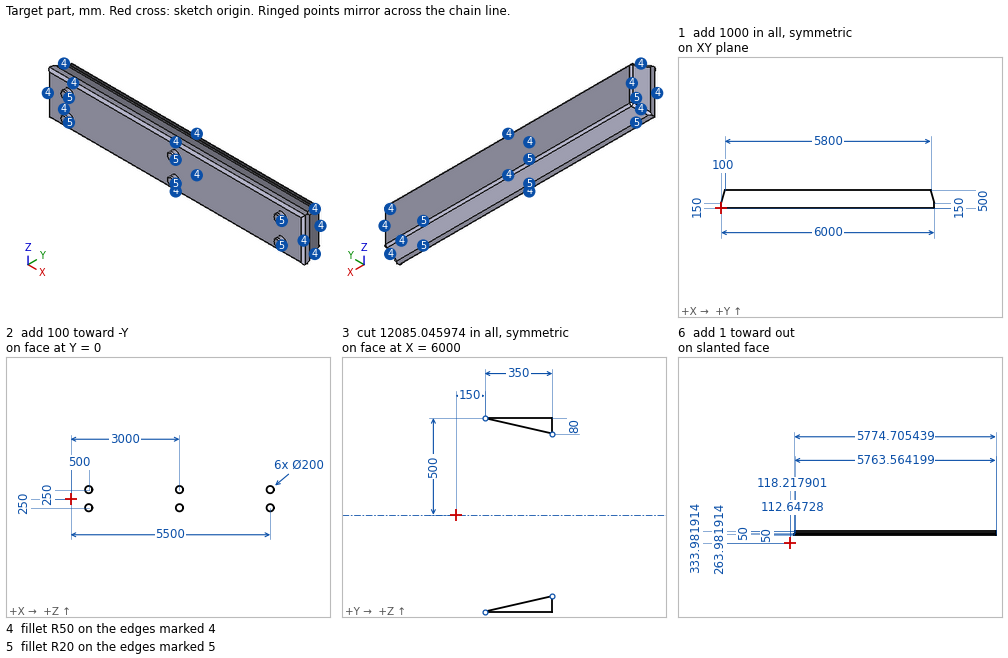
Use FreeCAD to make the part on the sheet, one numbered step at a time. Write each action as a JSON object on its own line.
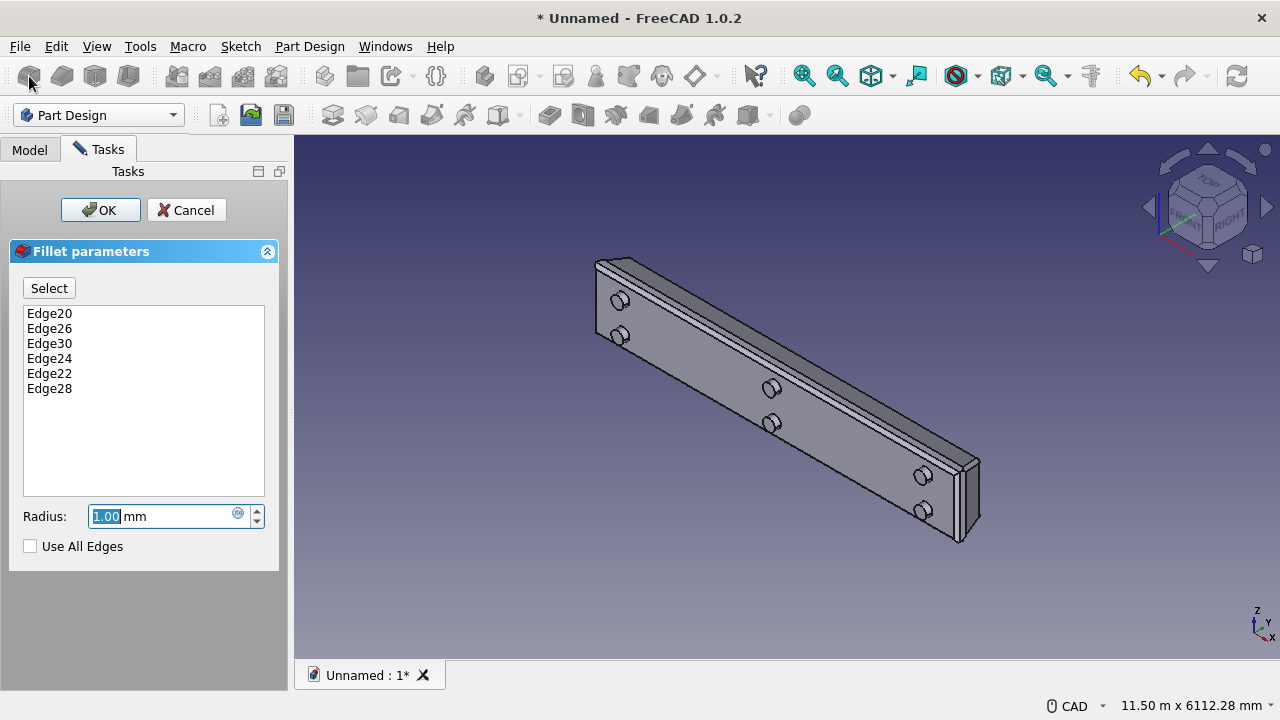
{"action": "type", "text": "20"}
{"action": "key", "text": "Tab"}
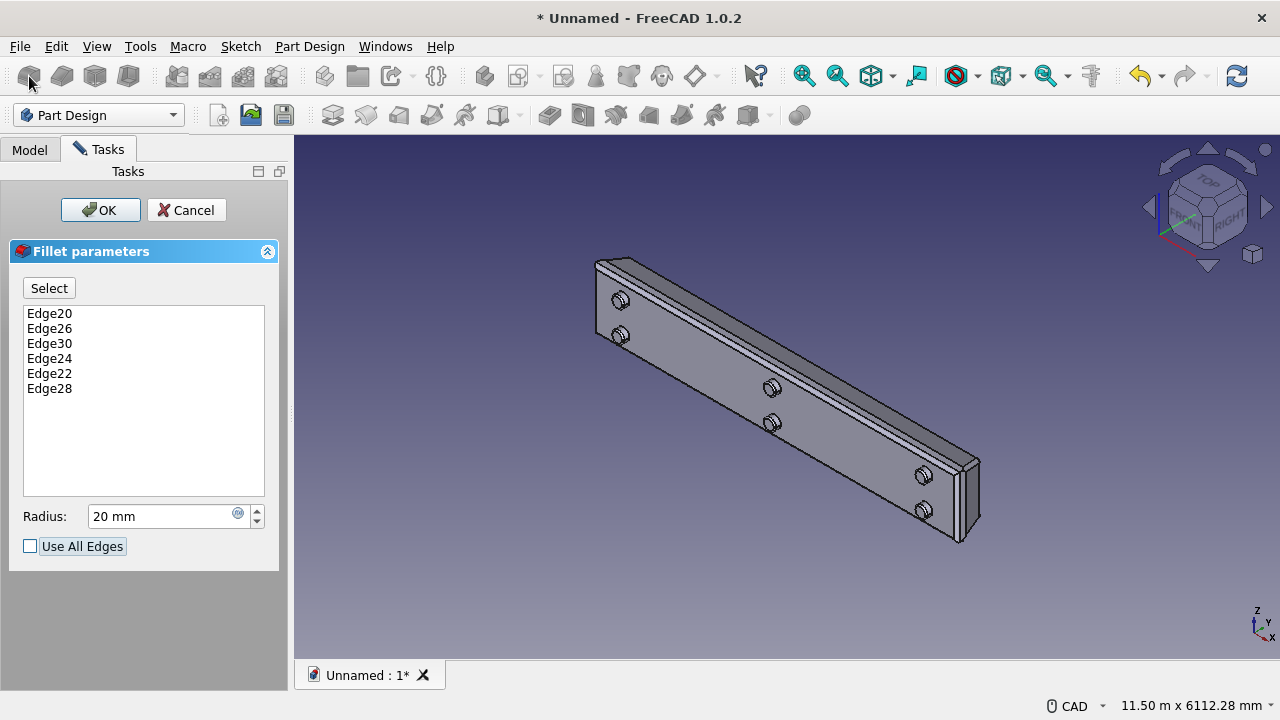
{"action": "left_click", "coordinate": [101, 210]}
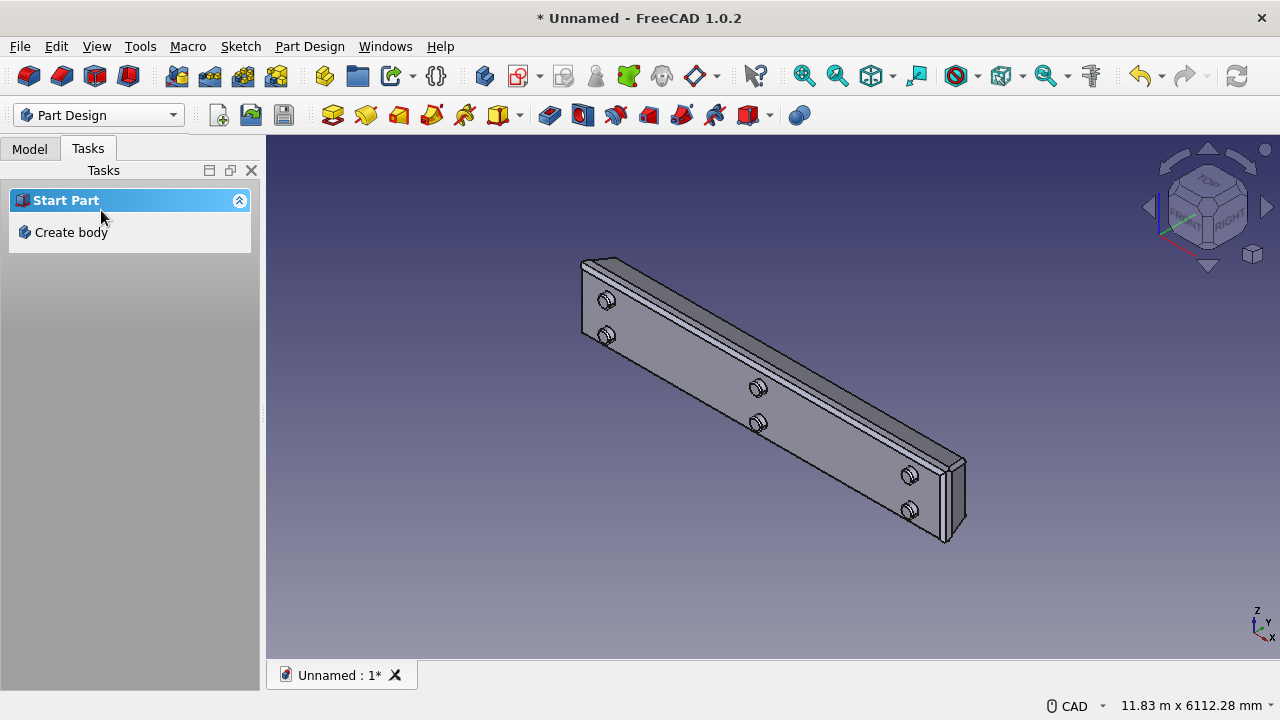
{"action": "key", "text": "2"}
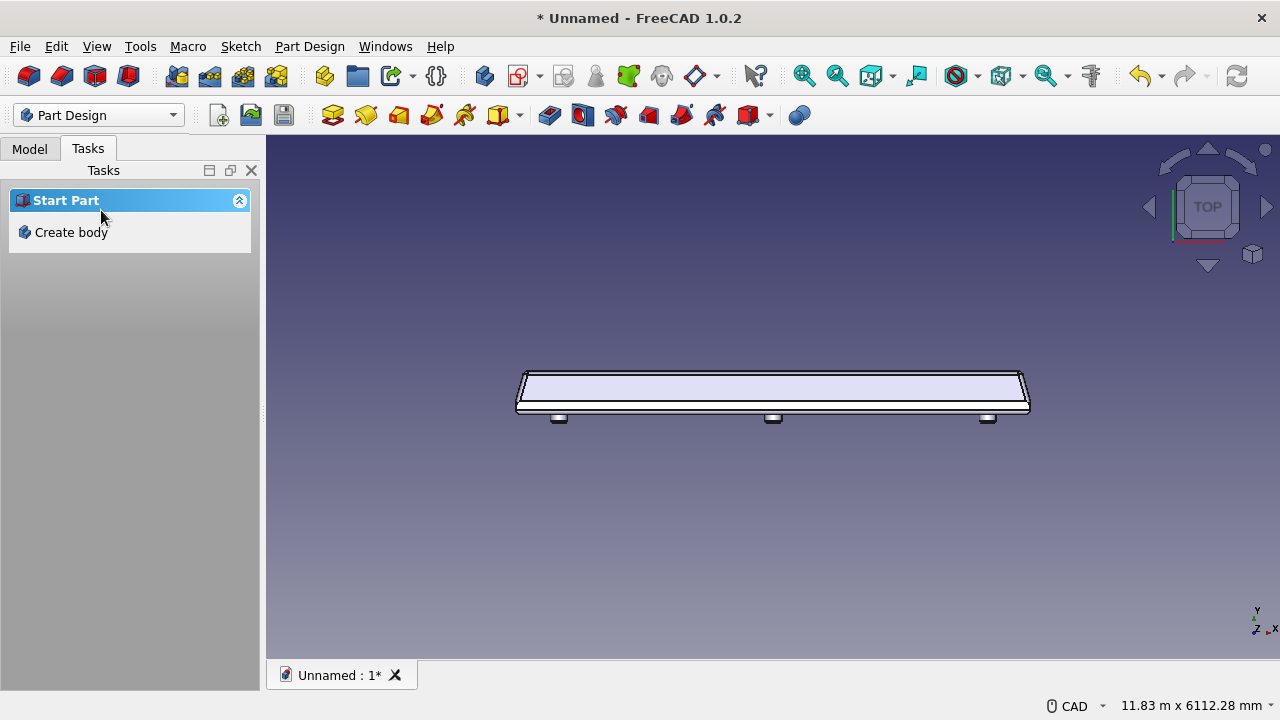
{"action": "left_click", "coordinate": [990, 387]}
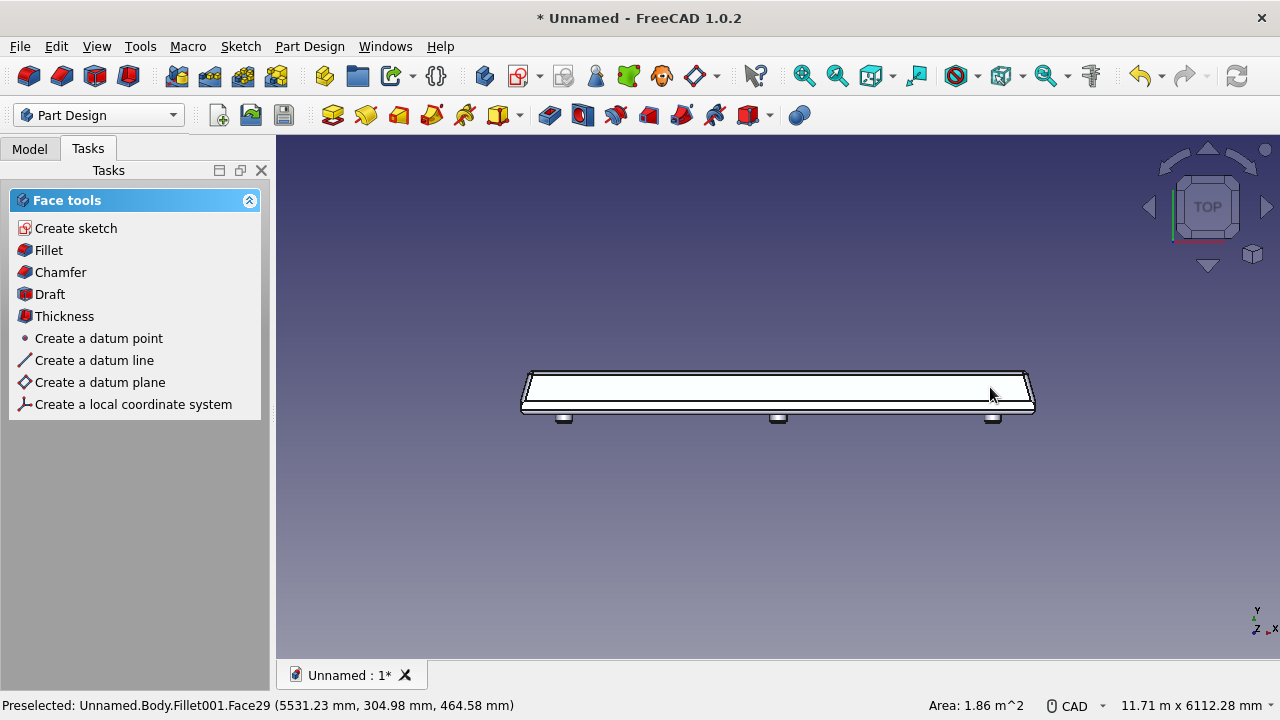
{"action": "left_click", "coordinate": [518, 76]}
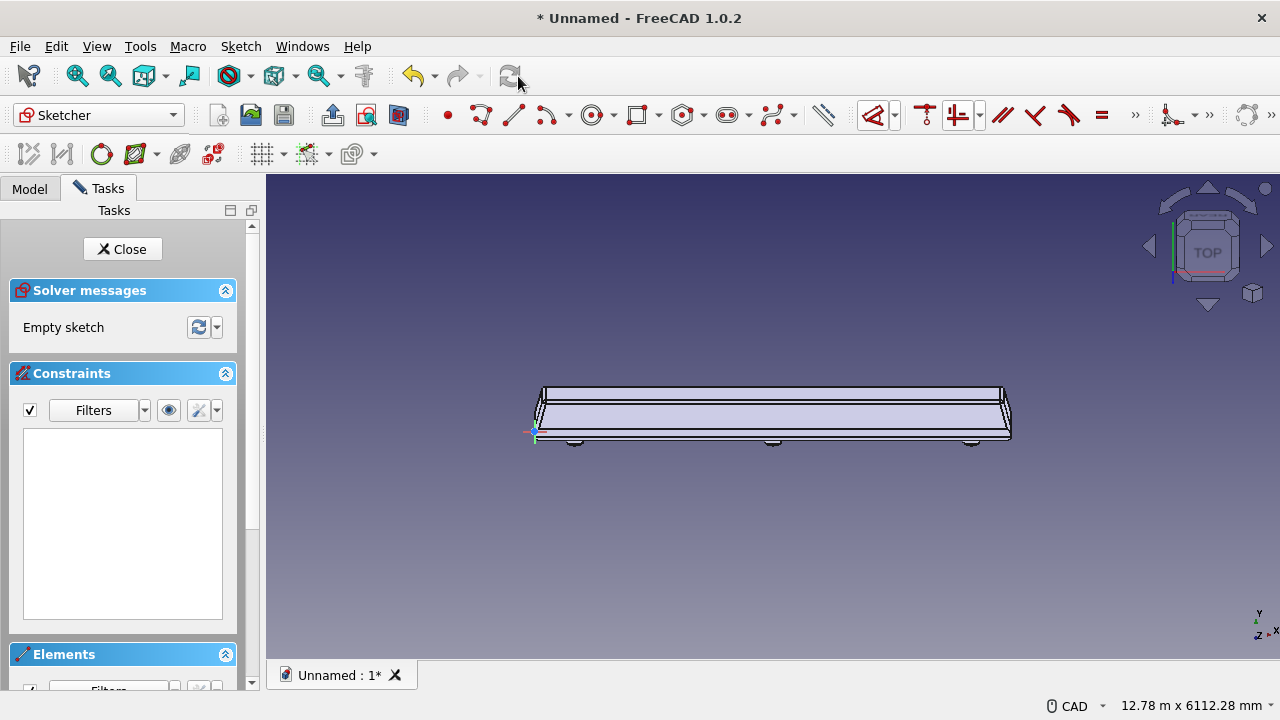
{"action": "left_click", "coordinate": [636, 116]}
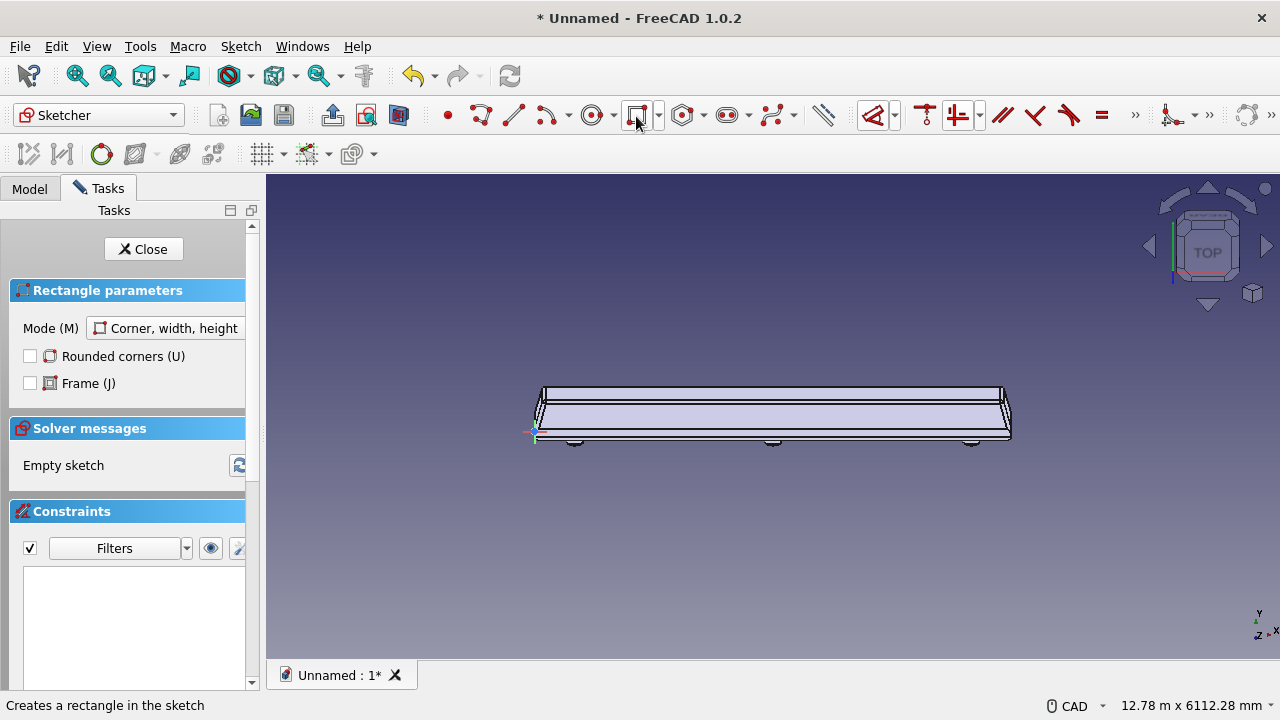
{"action": "scroll", "coordinate": [544, 405], "scroll_direction": "up", "scroll_amount": 7}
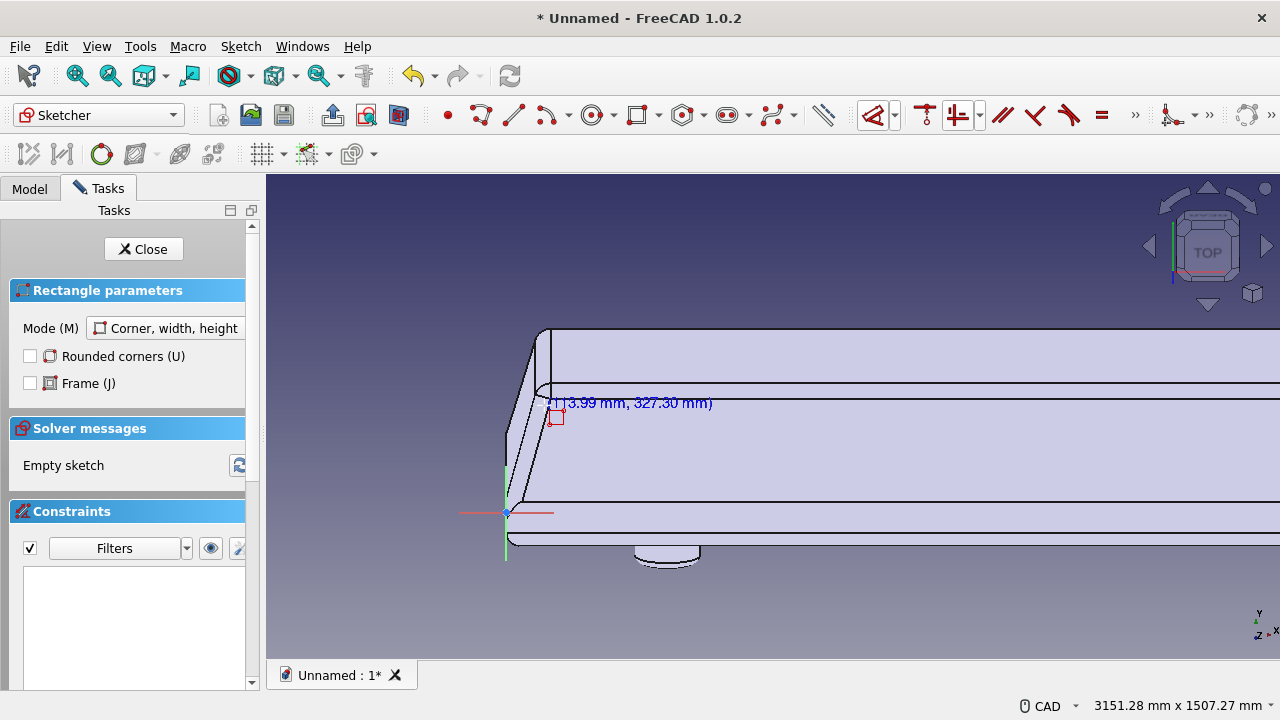
{"action": "left_click", "coordinate": [545, 405]}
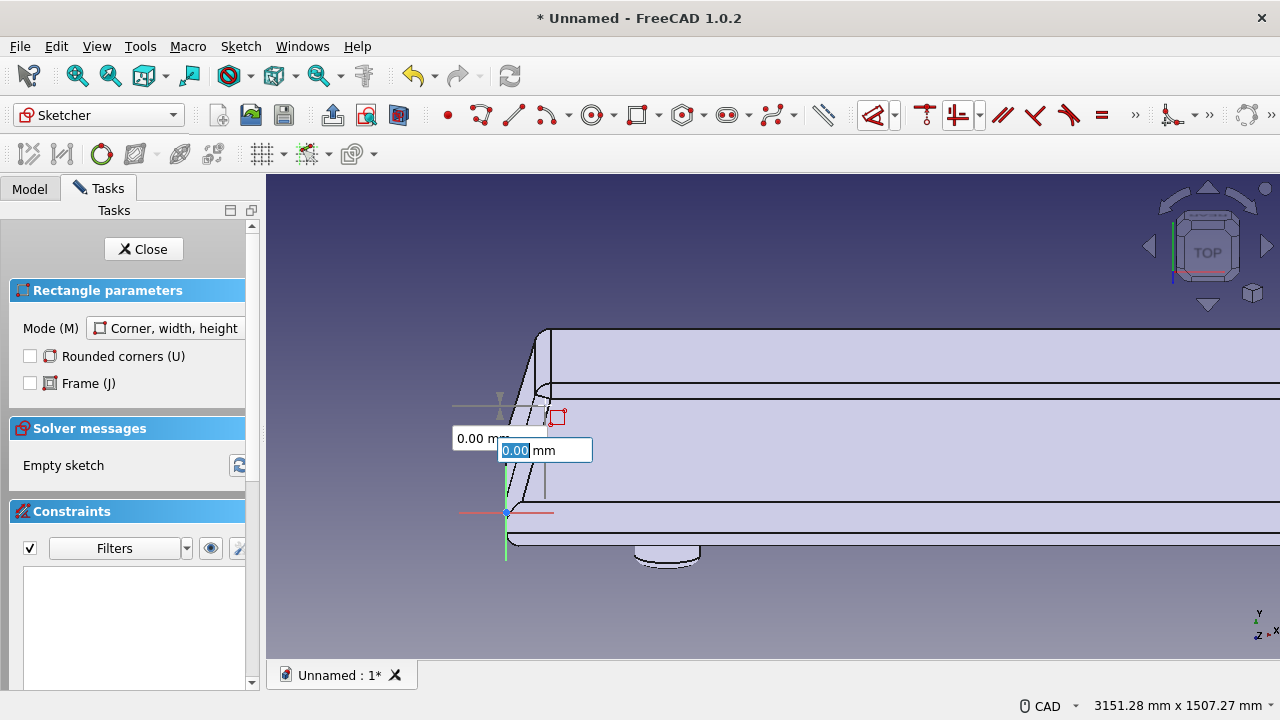
{"action": "scroll", "coordinate": [382, 398], "scroll_direction": "down", "scroll_amount": 6}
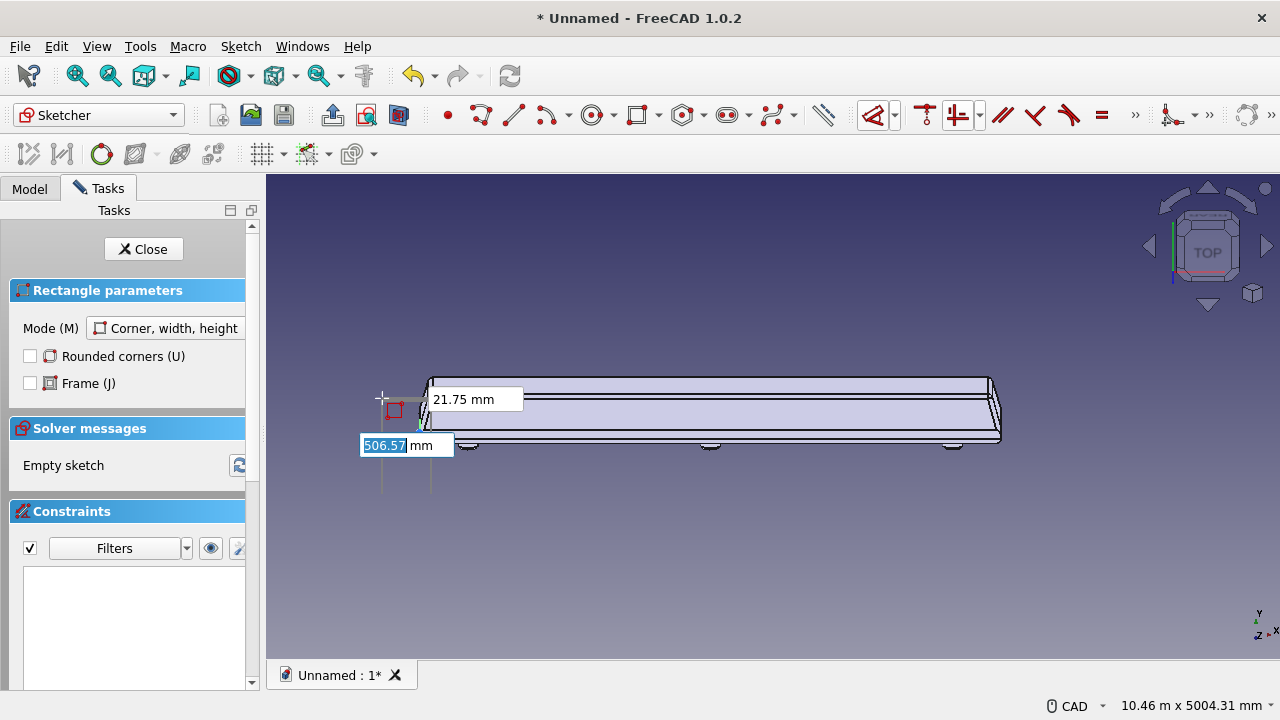
{"action": "left_click", "coordinate": [990, 405]}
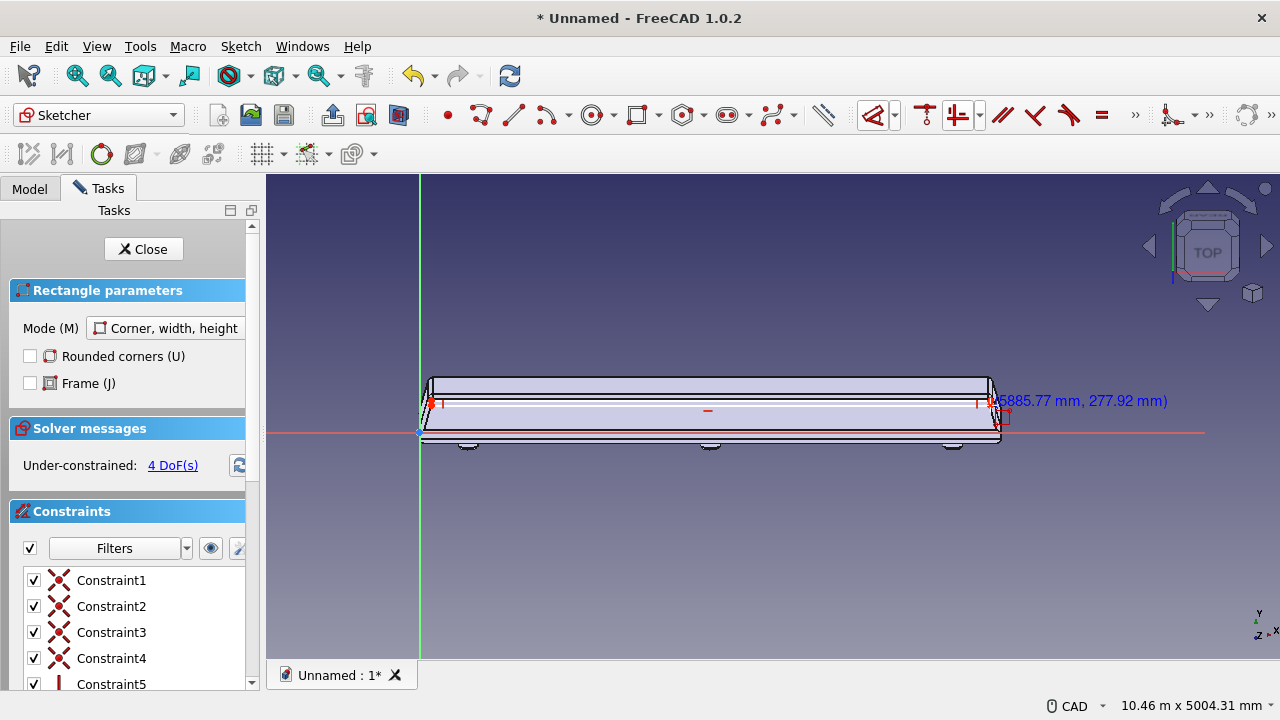
{"action": "scroll", "coordinate": [430, 407], "scroll_direction": "up", "scroll_amount": 11}